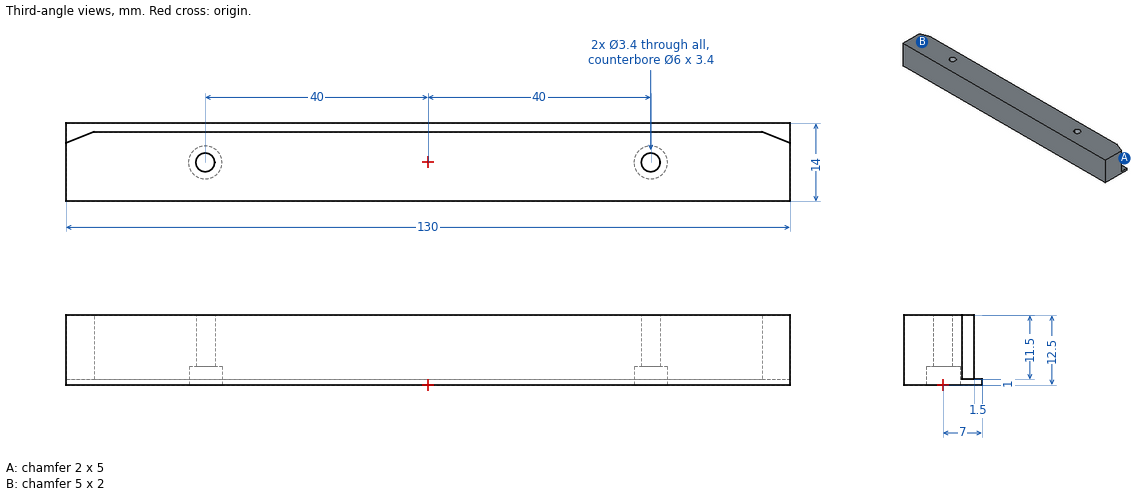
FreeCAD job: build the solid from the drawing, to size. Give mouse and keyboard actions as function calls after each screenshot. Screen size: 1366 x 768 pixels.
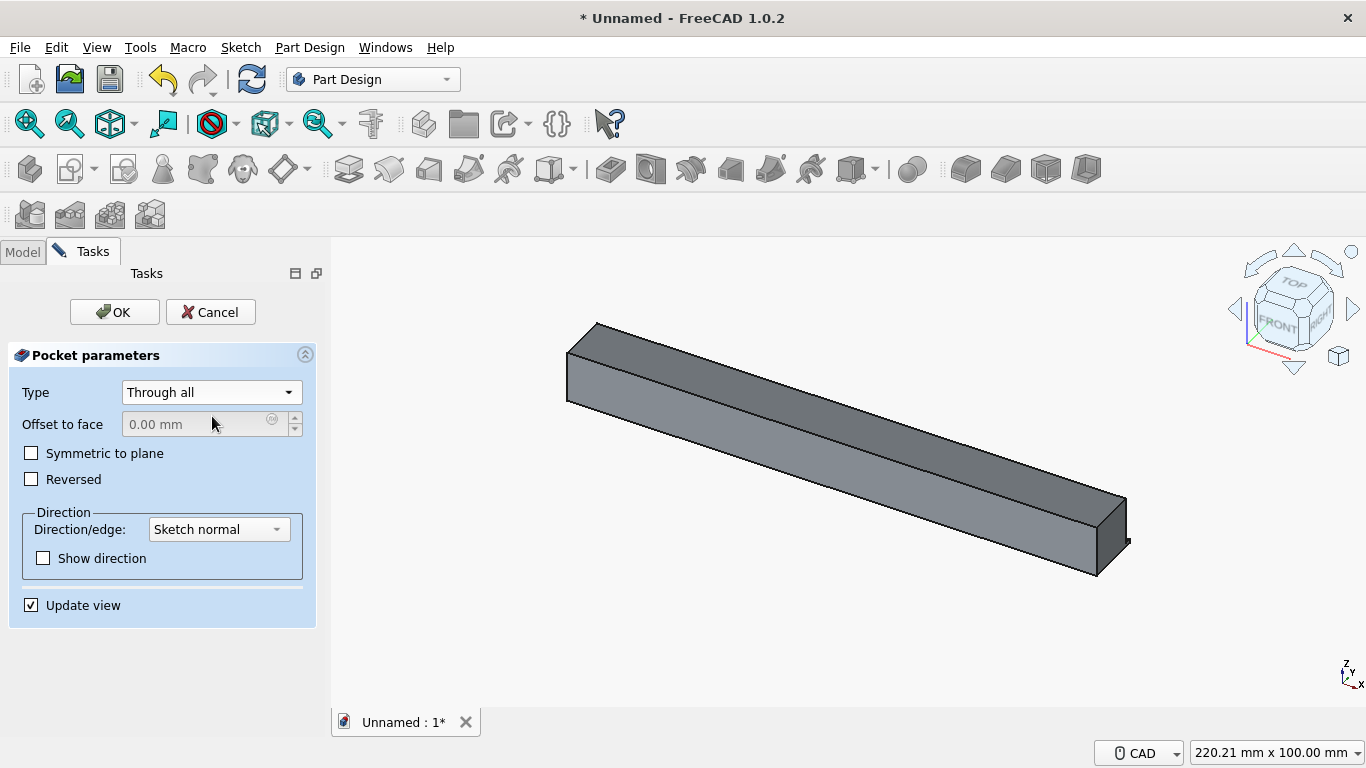
click(115, 312)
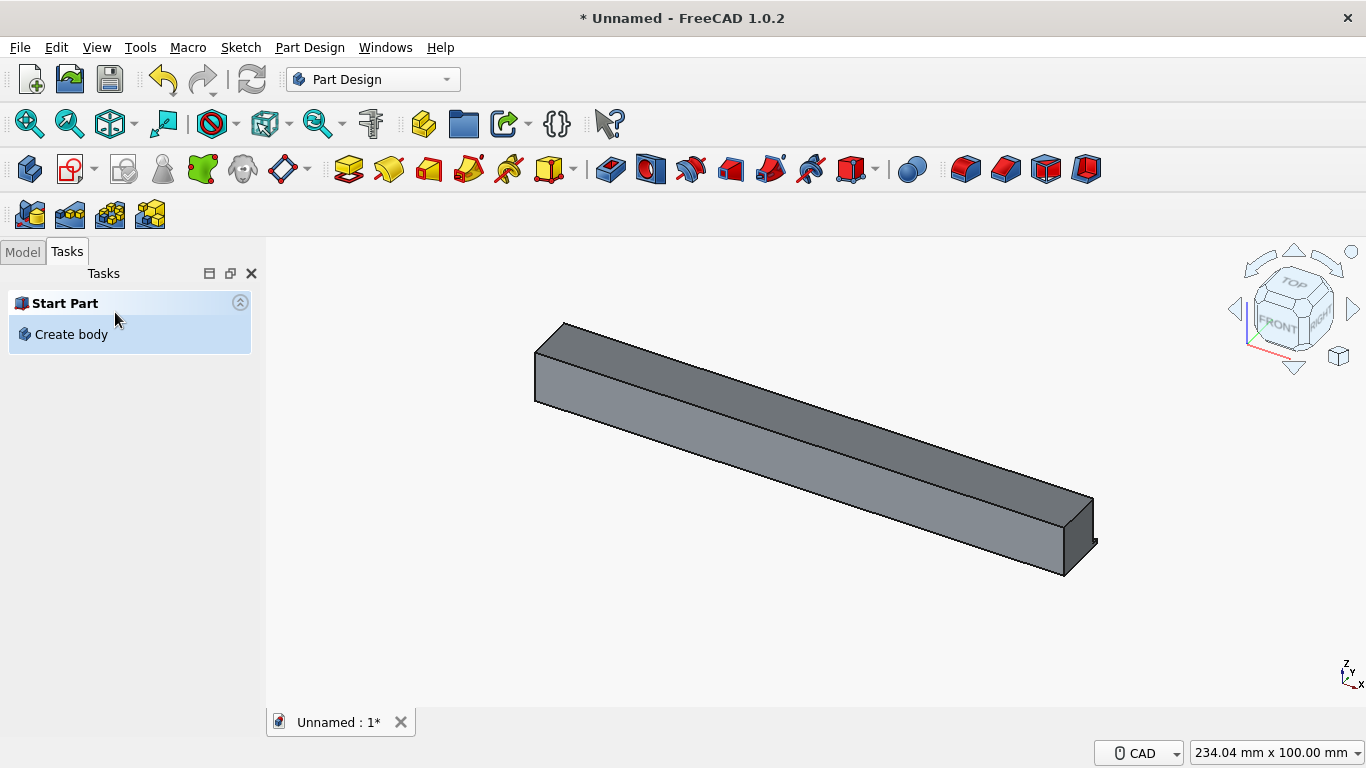
key(0)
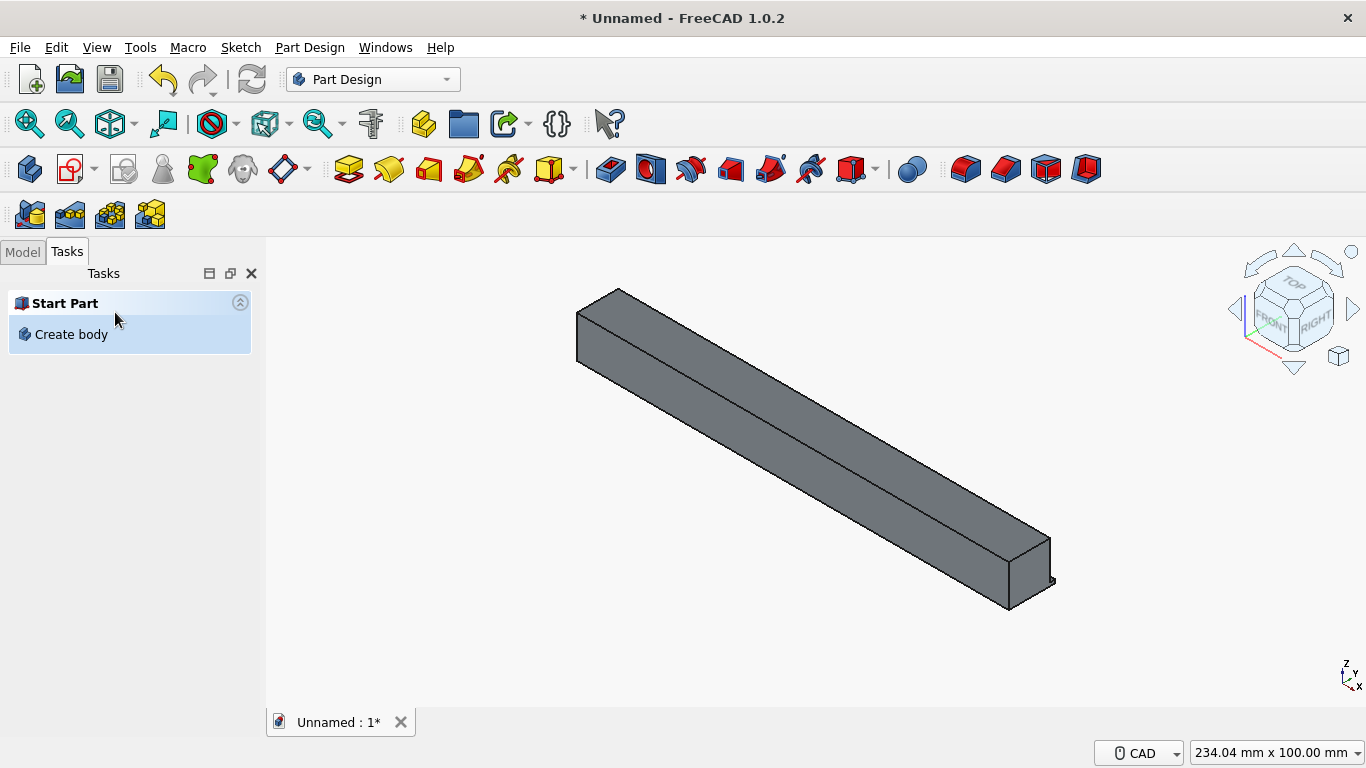
key(2)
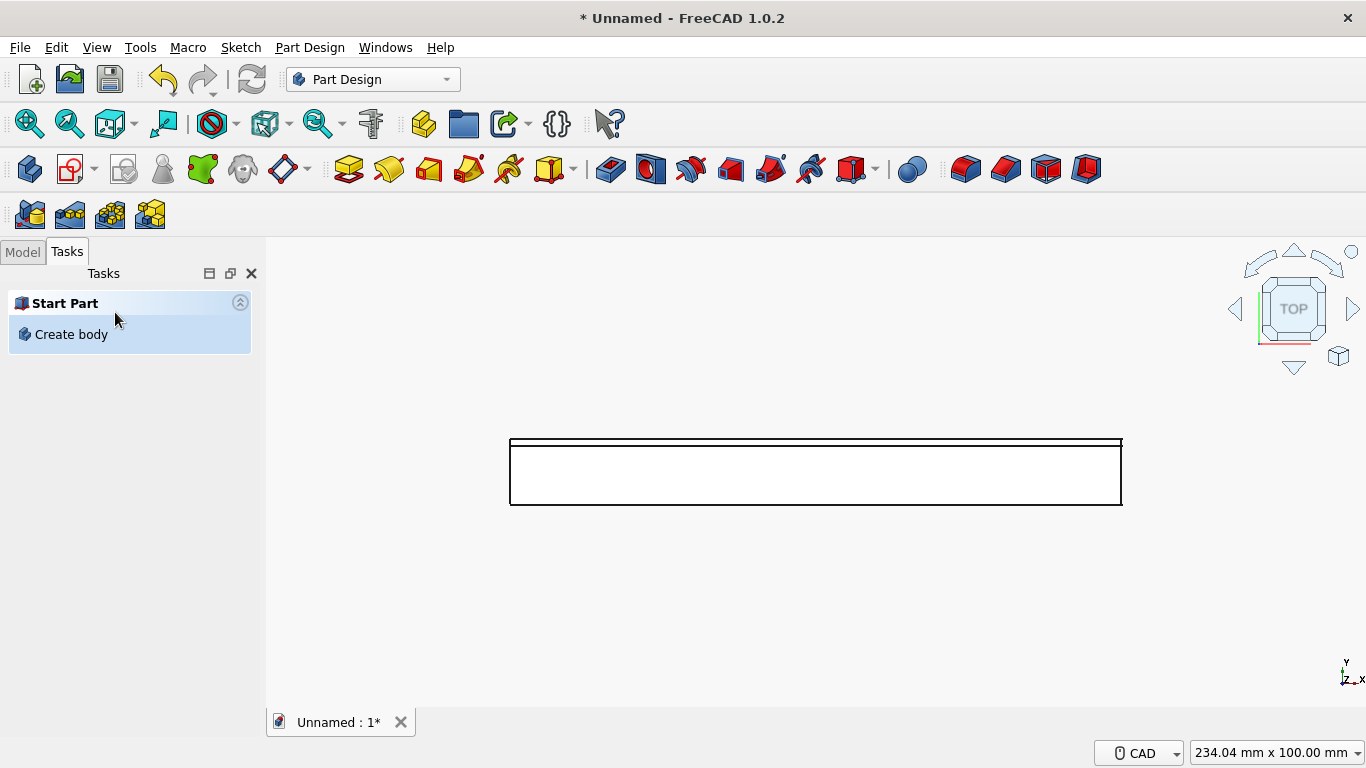
key(1)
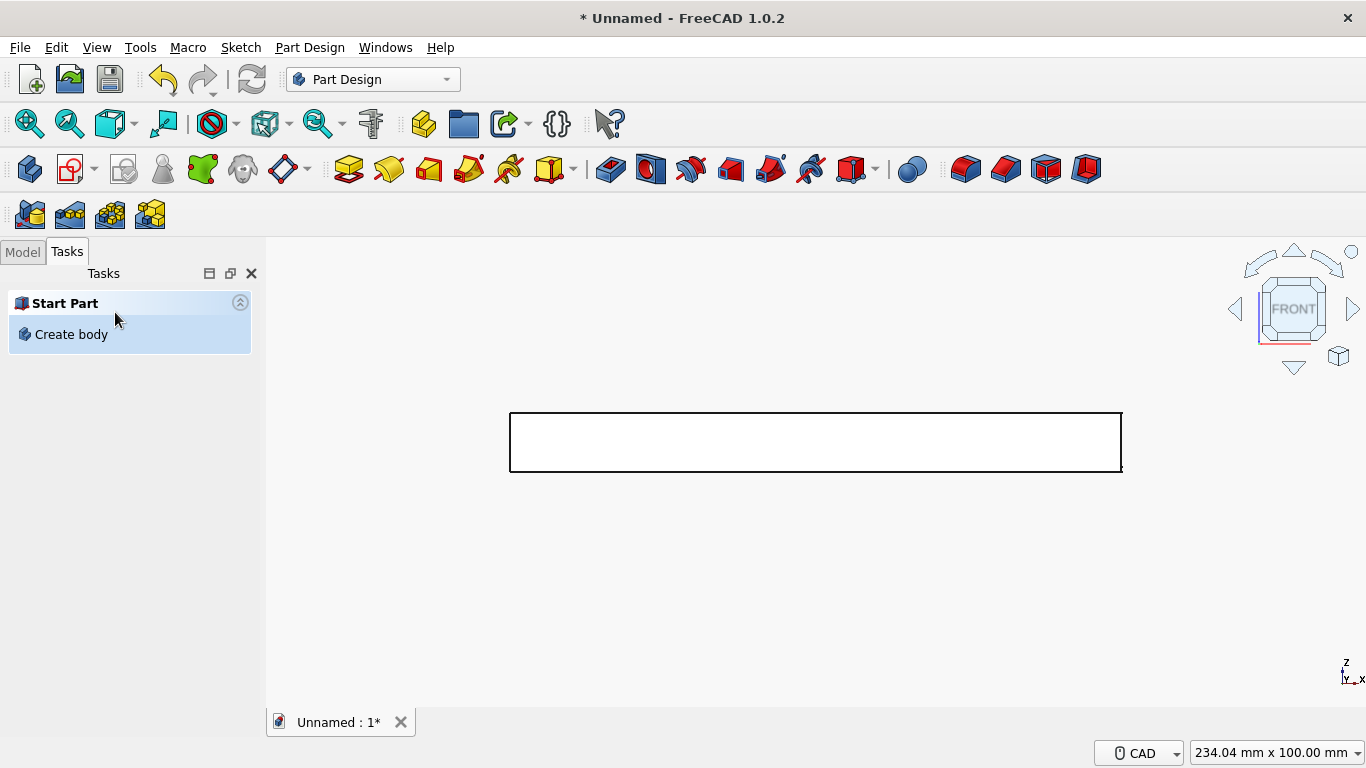
key(3)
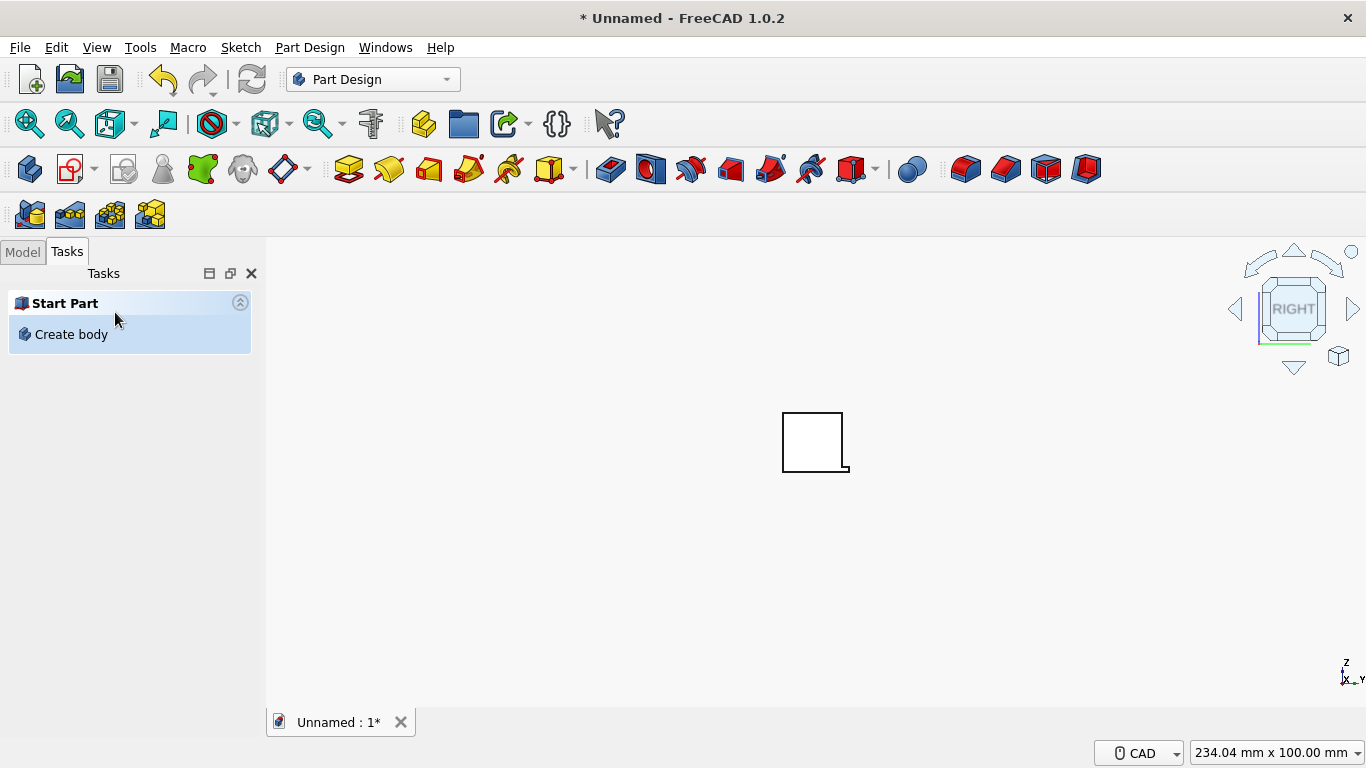
click(30, 124)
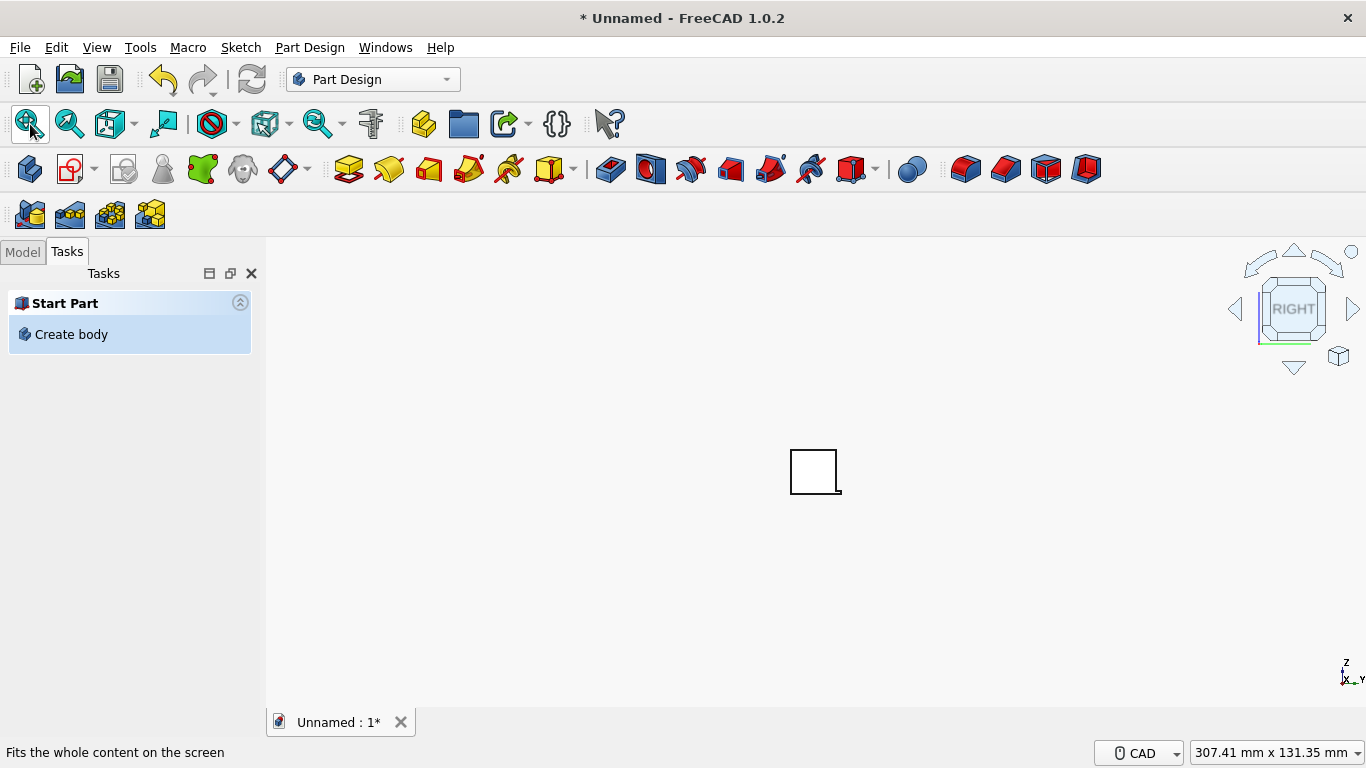
click(836, 469)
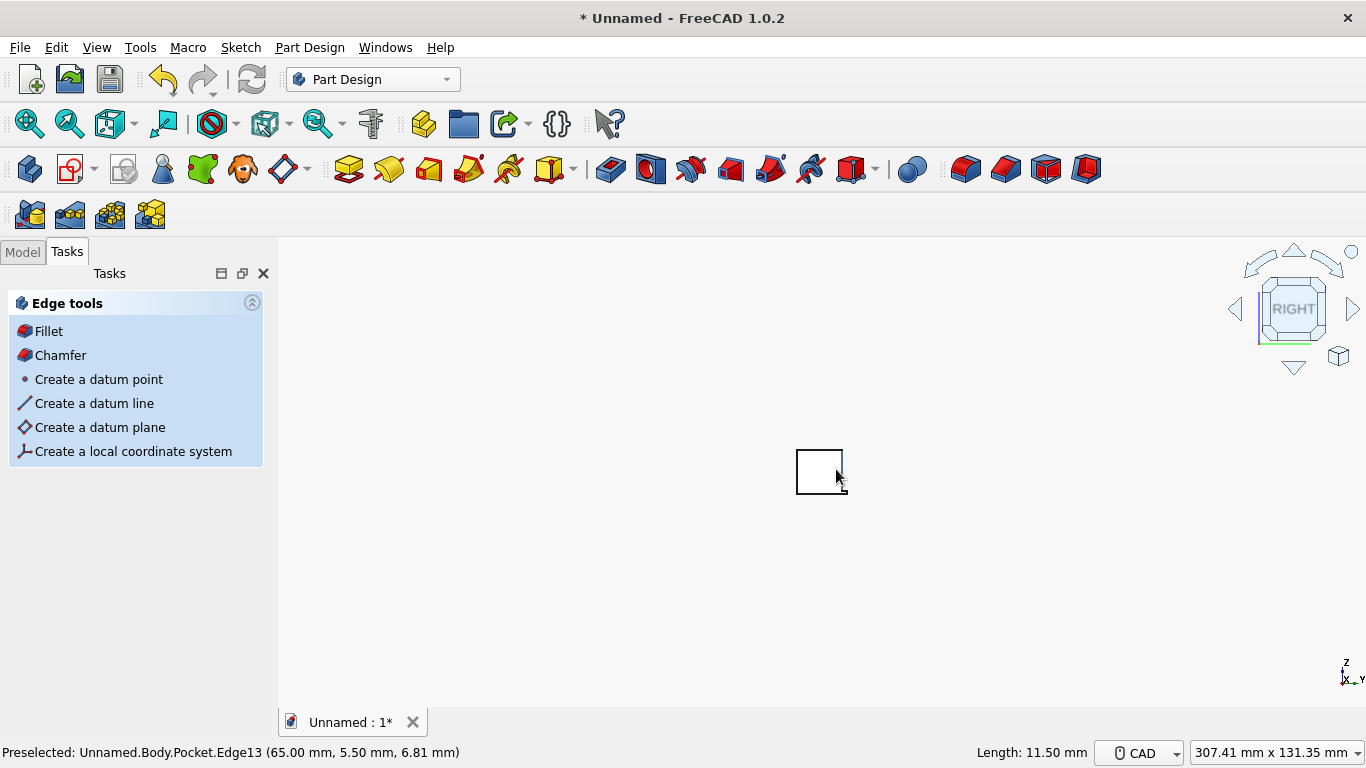
click(1006, 170)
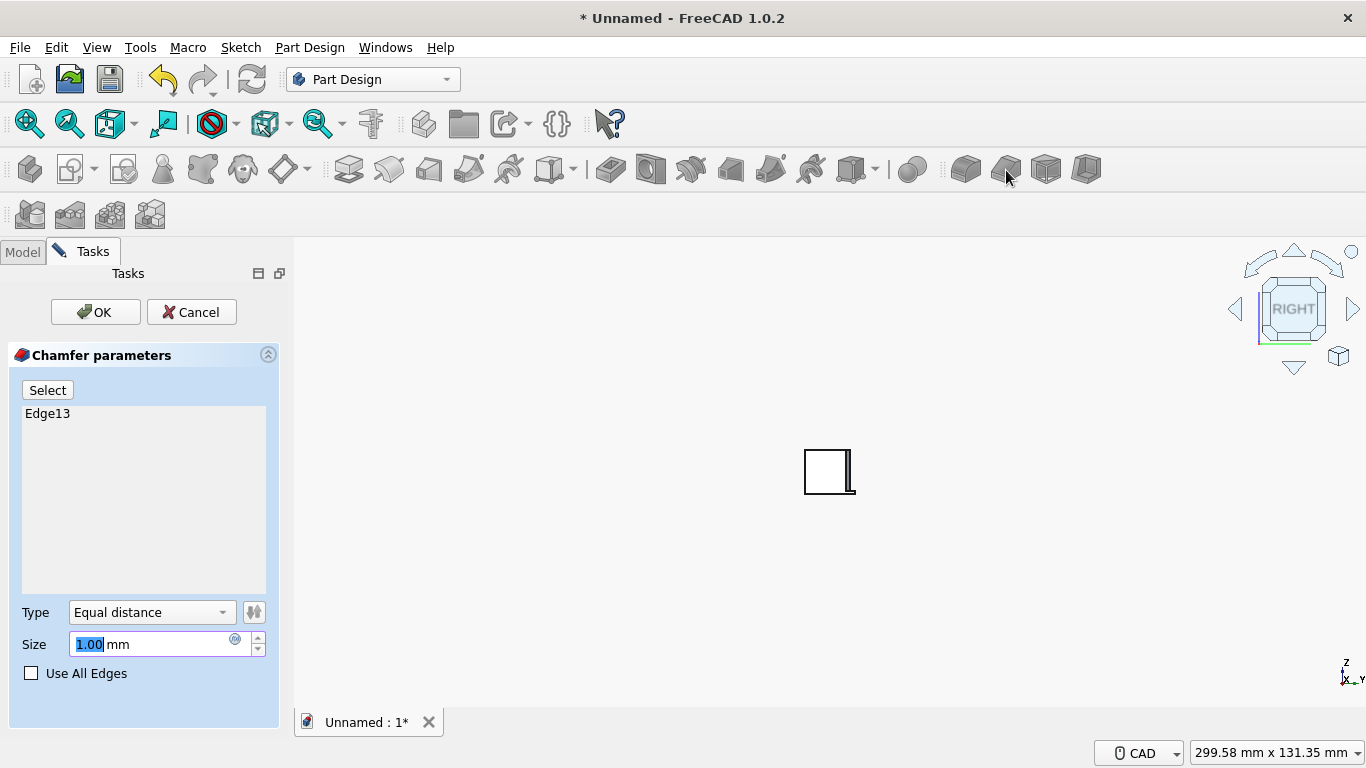
text(2)
key(Tab)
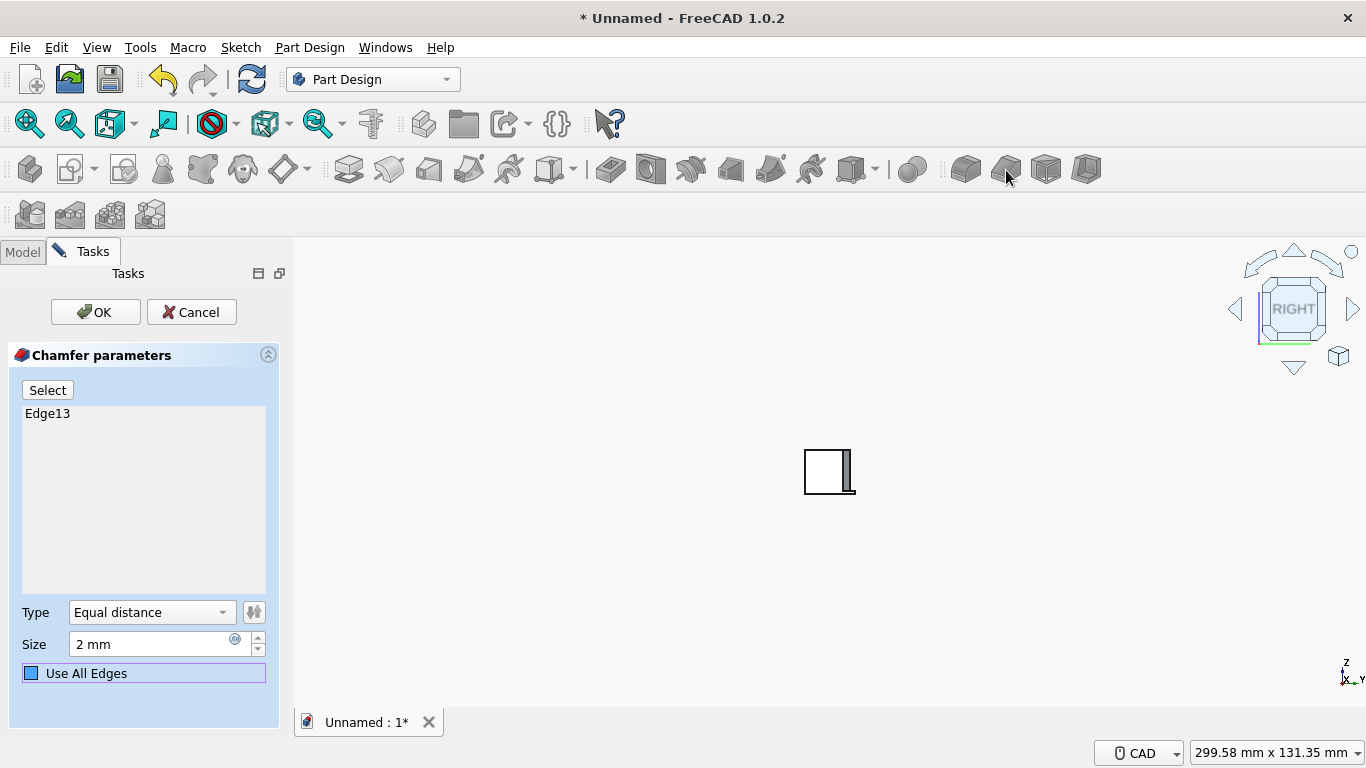
click(153, 612)